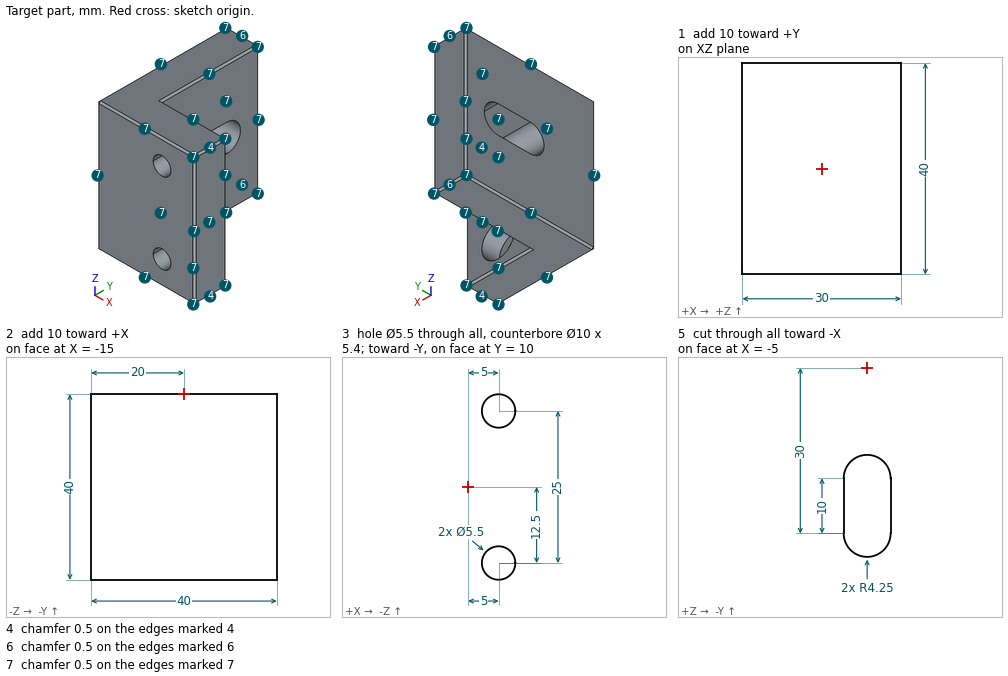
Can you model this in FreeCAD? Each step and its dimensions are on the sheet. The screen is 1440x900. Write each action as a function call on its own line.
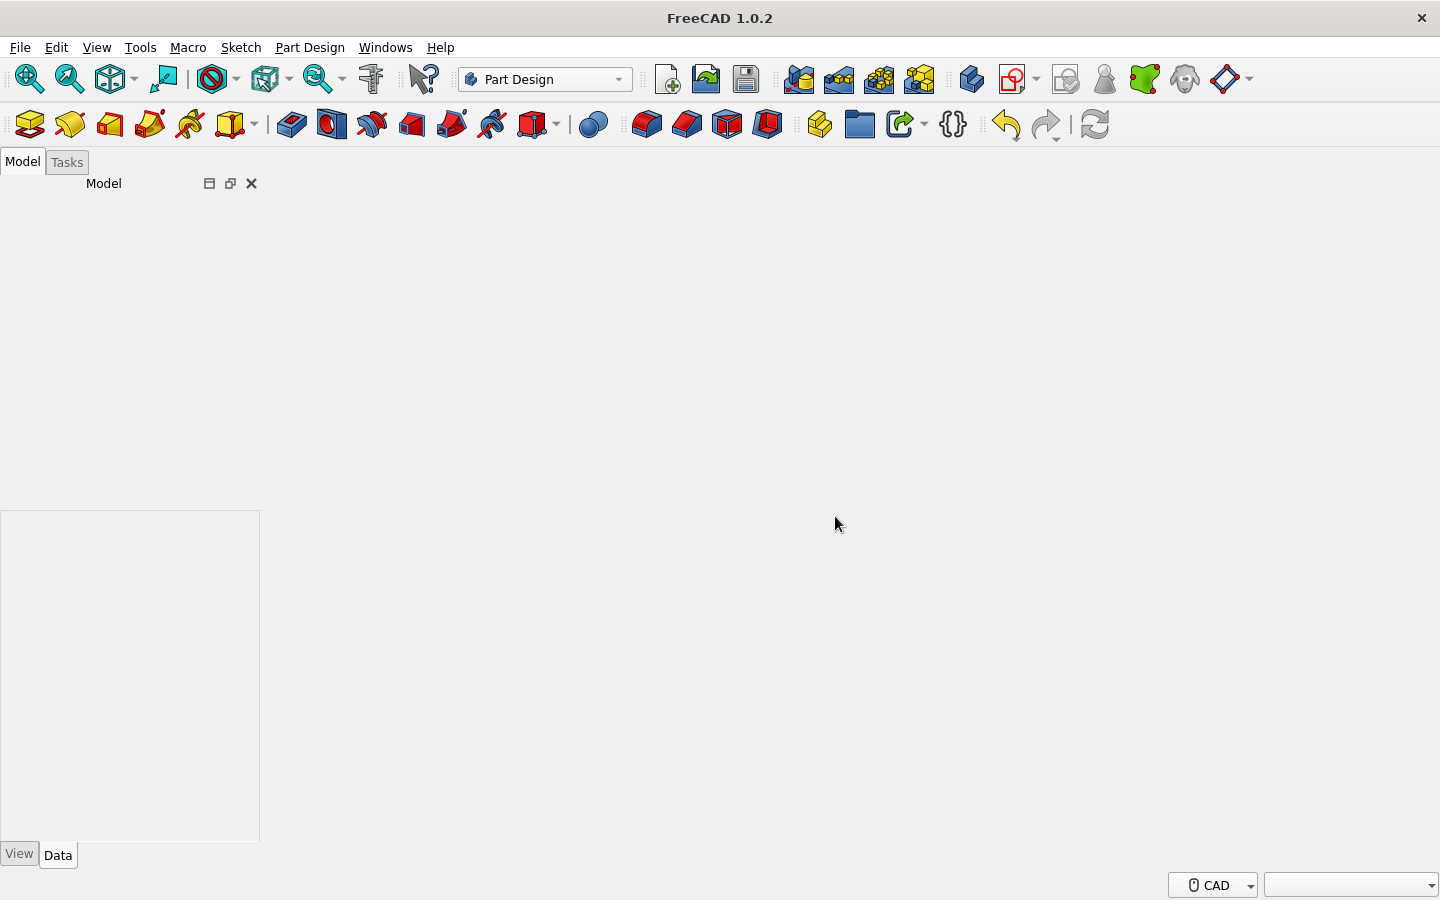
click(666, 80)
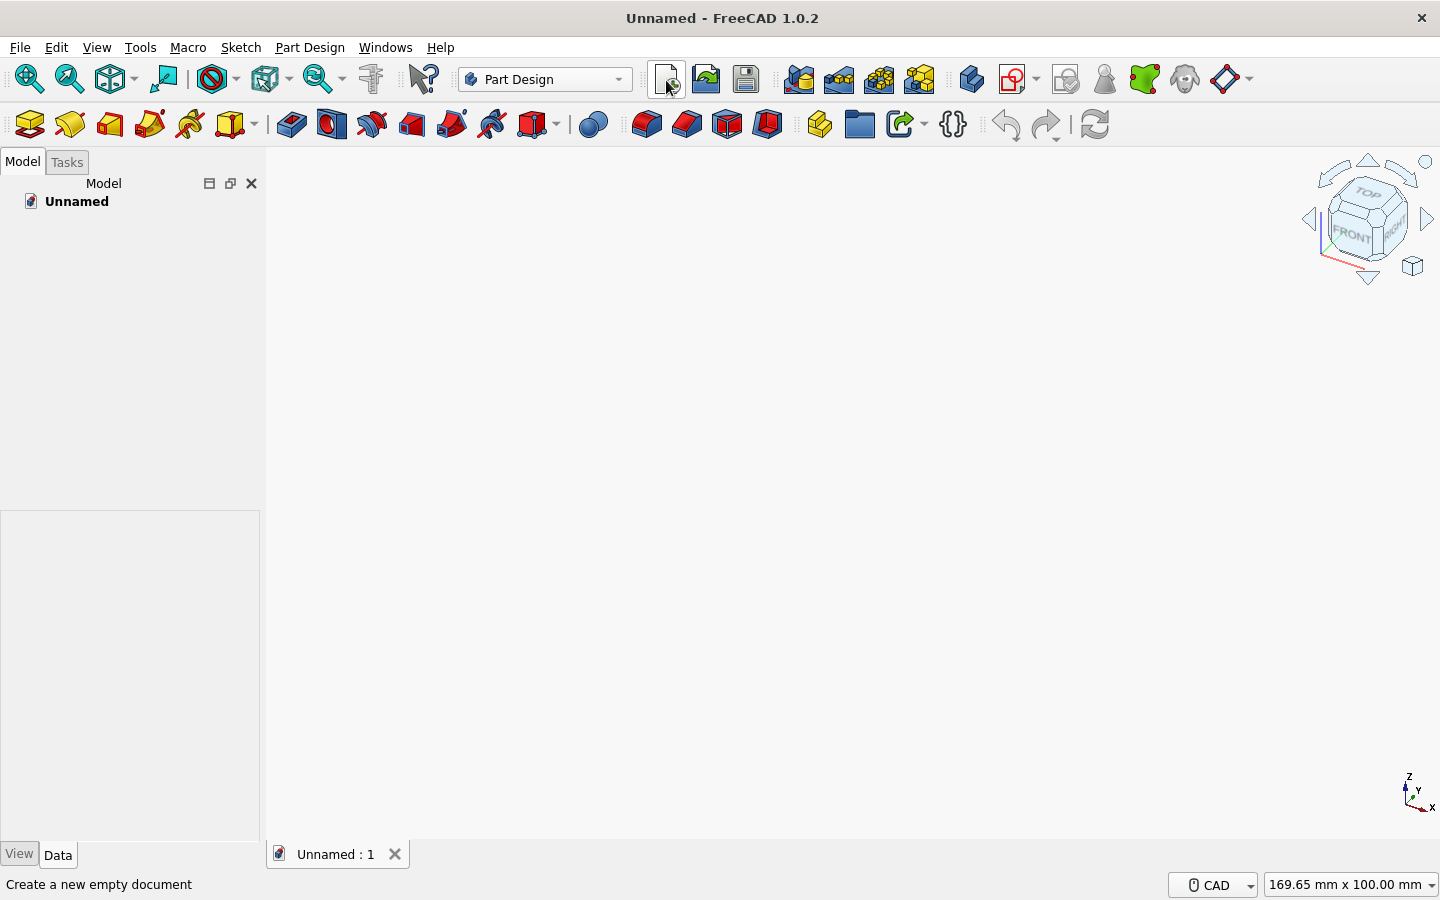
click(1012, 80)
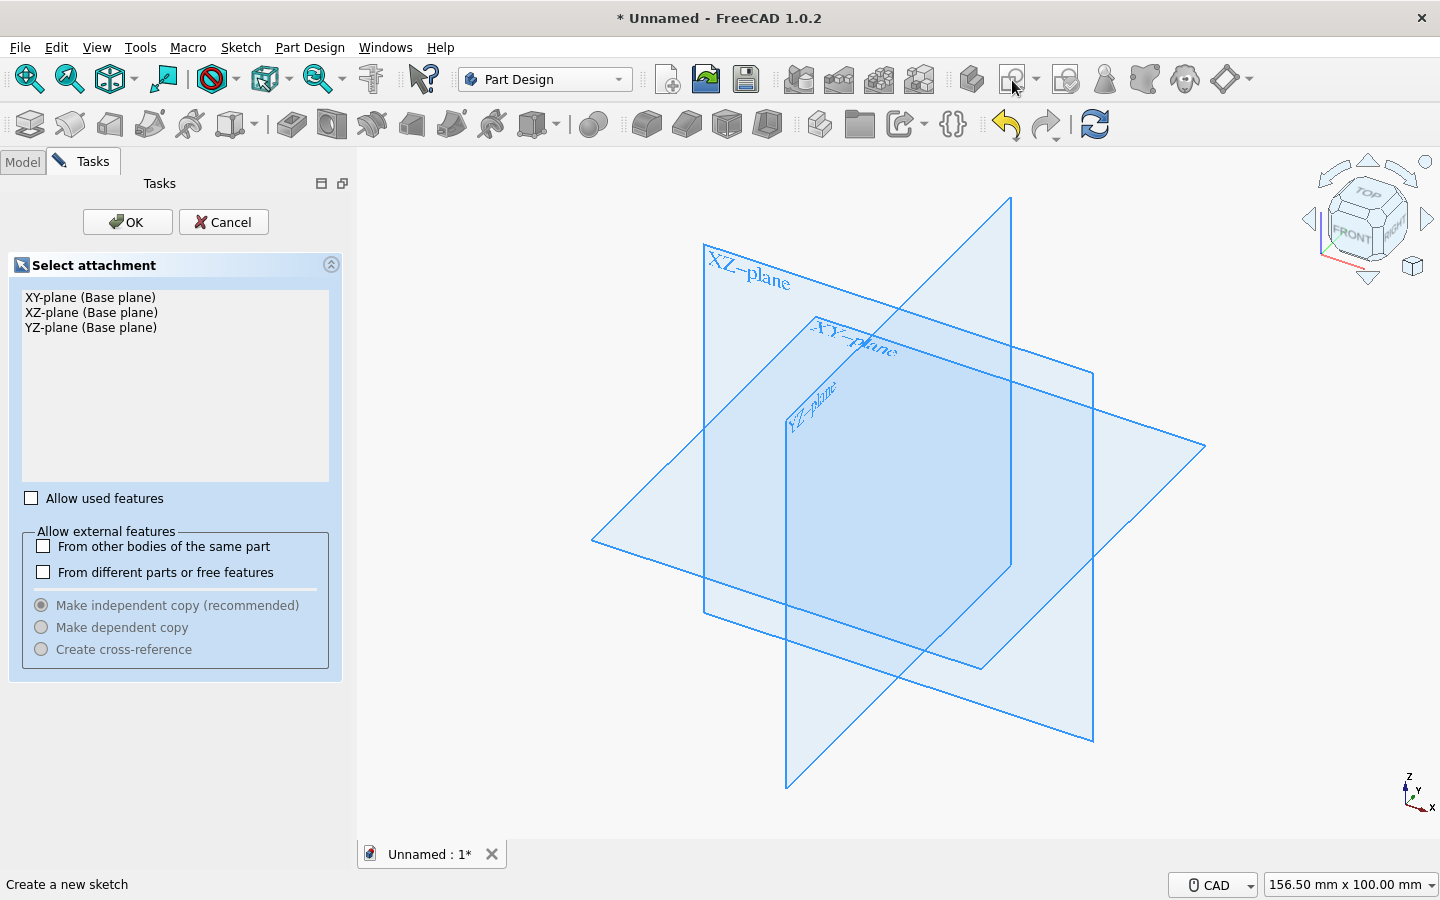
click(82, 312)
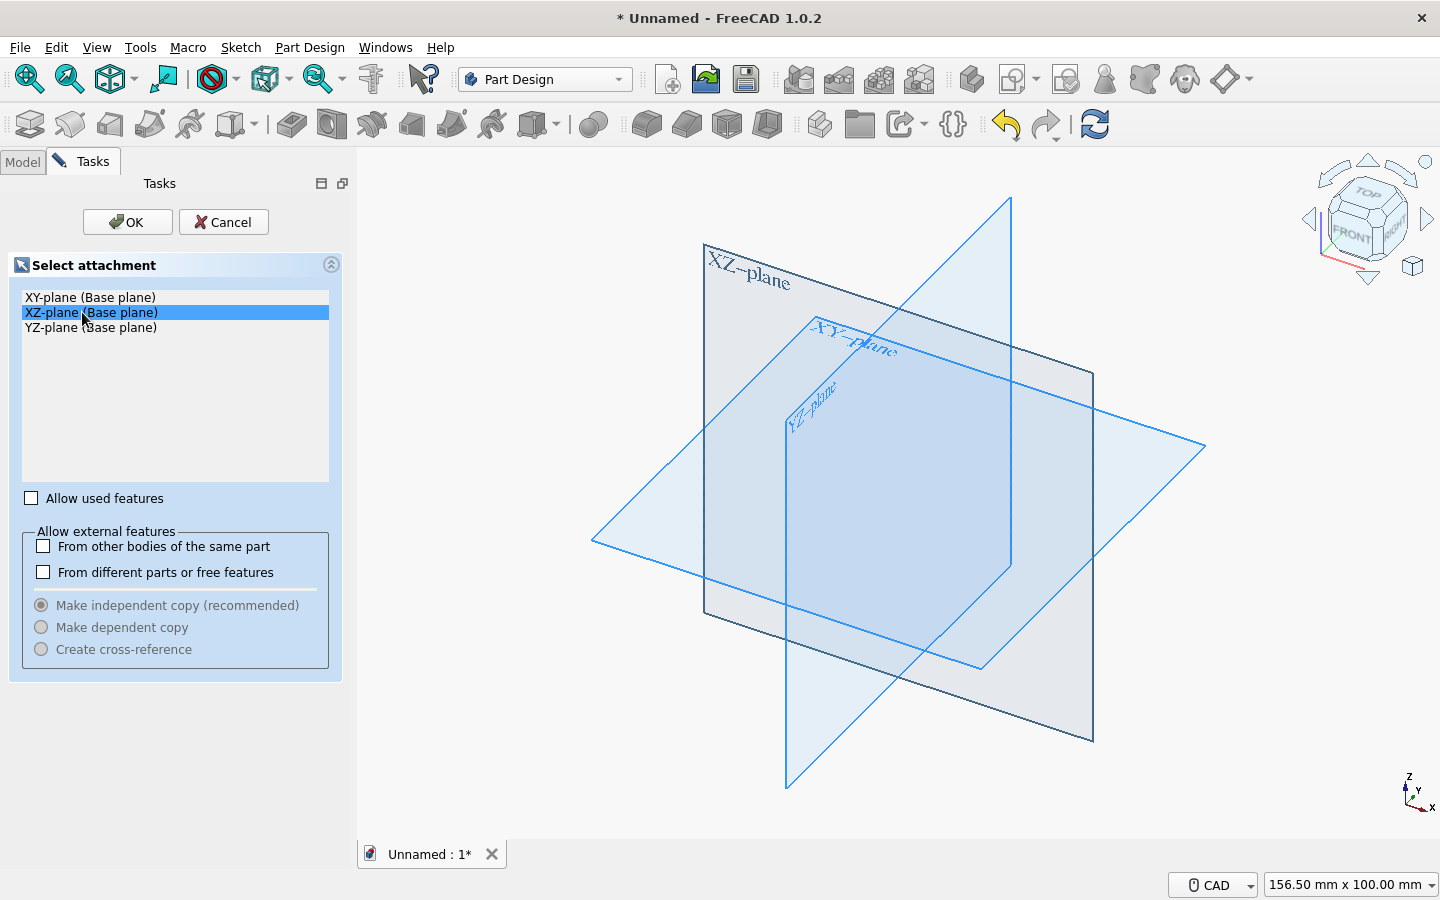
click(128, 222)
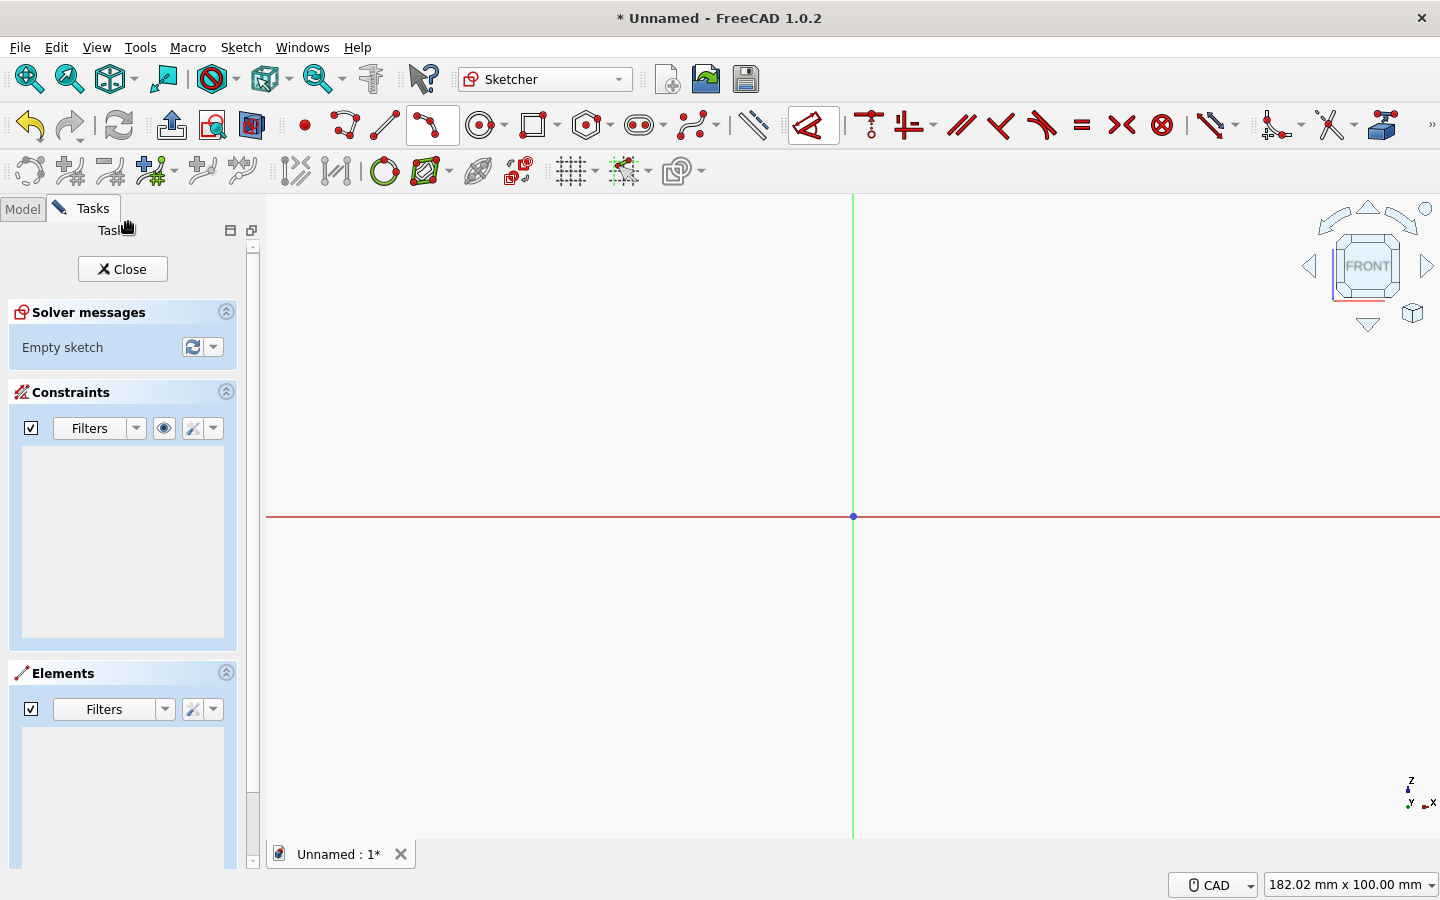
scroll(992, 517, up, 2)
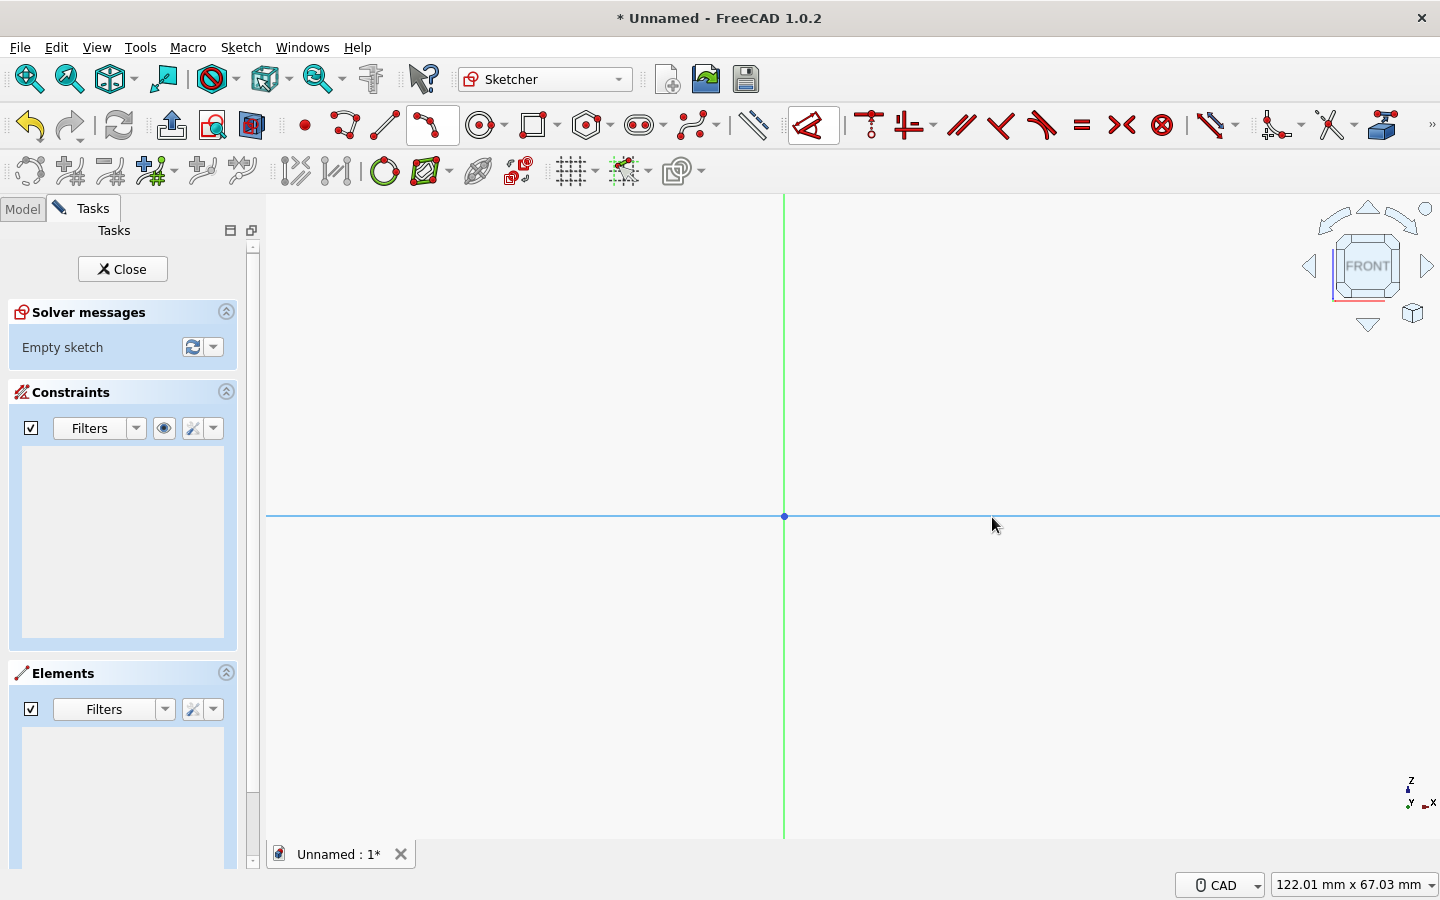
key(g)
key(v)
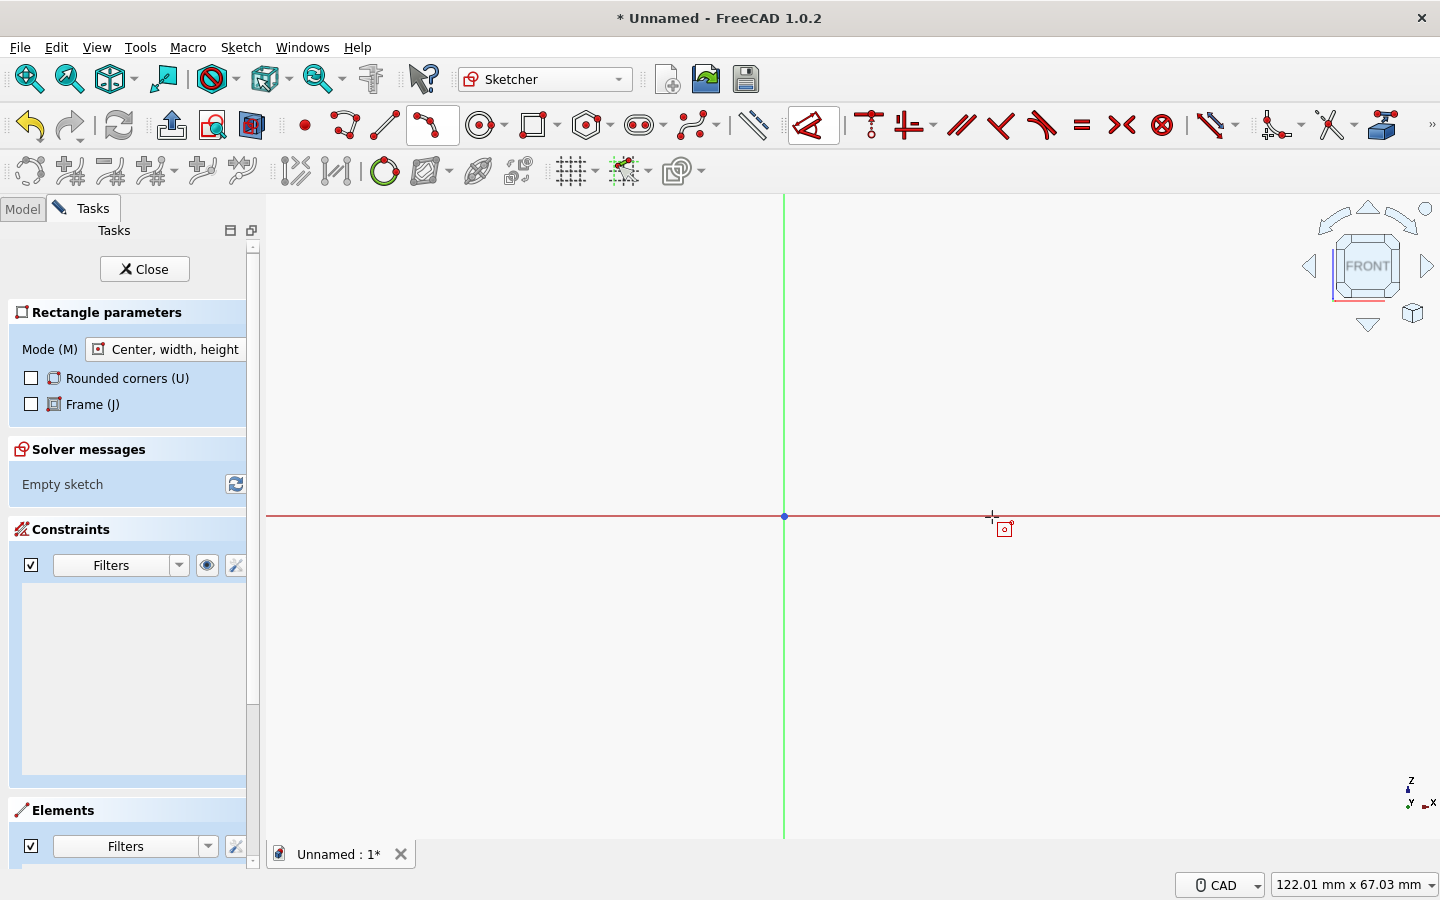
click(784, 516)
click(929, 324)
key(Escape)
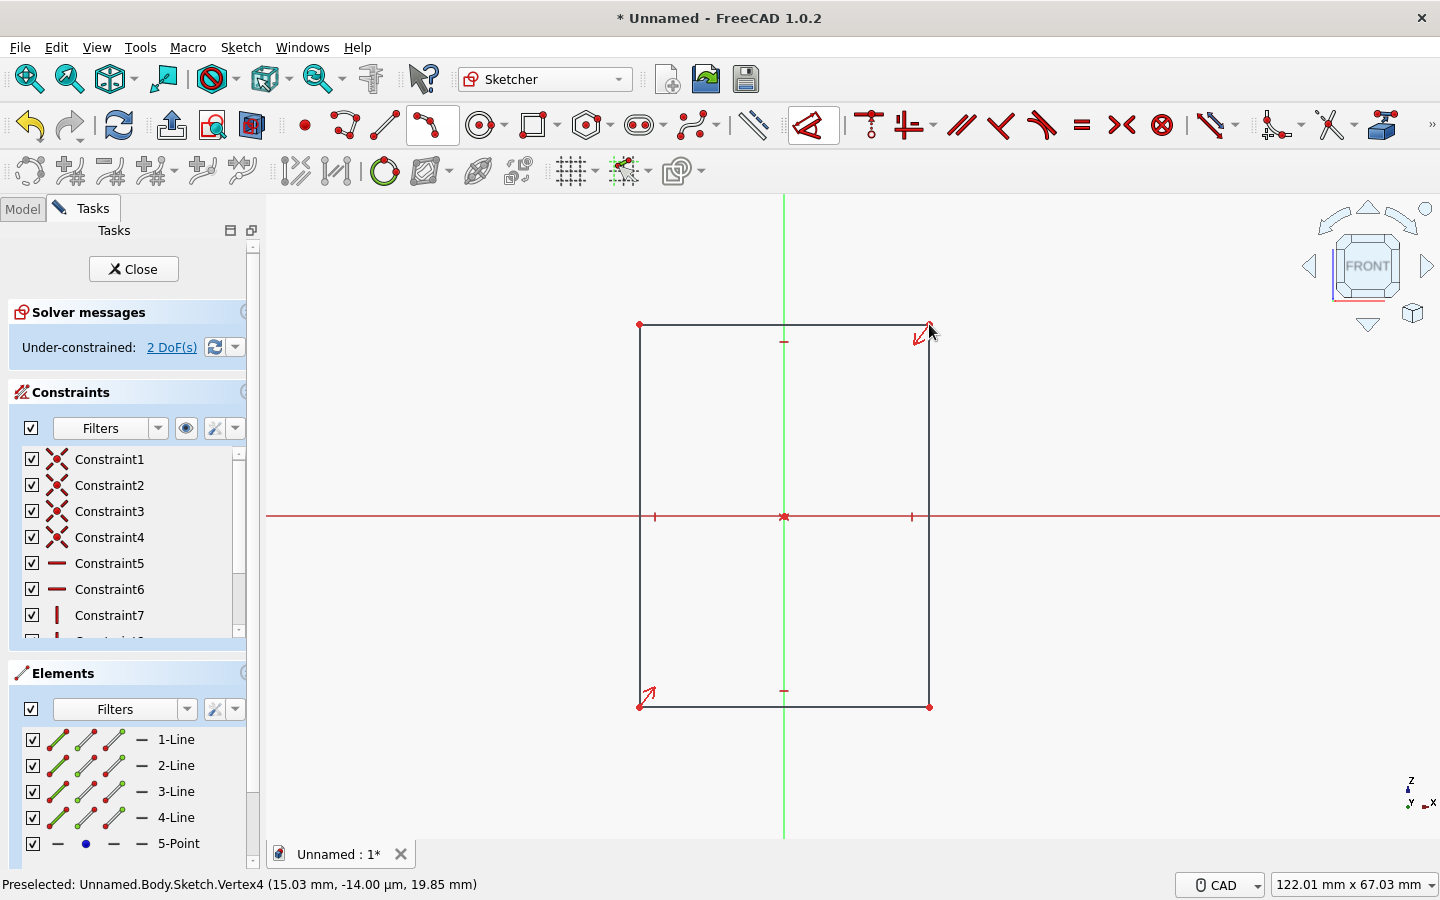
click(726, 707)